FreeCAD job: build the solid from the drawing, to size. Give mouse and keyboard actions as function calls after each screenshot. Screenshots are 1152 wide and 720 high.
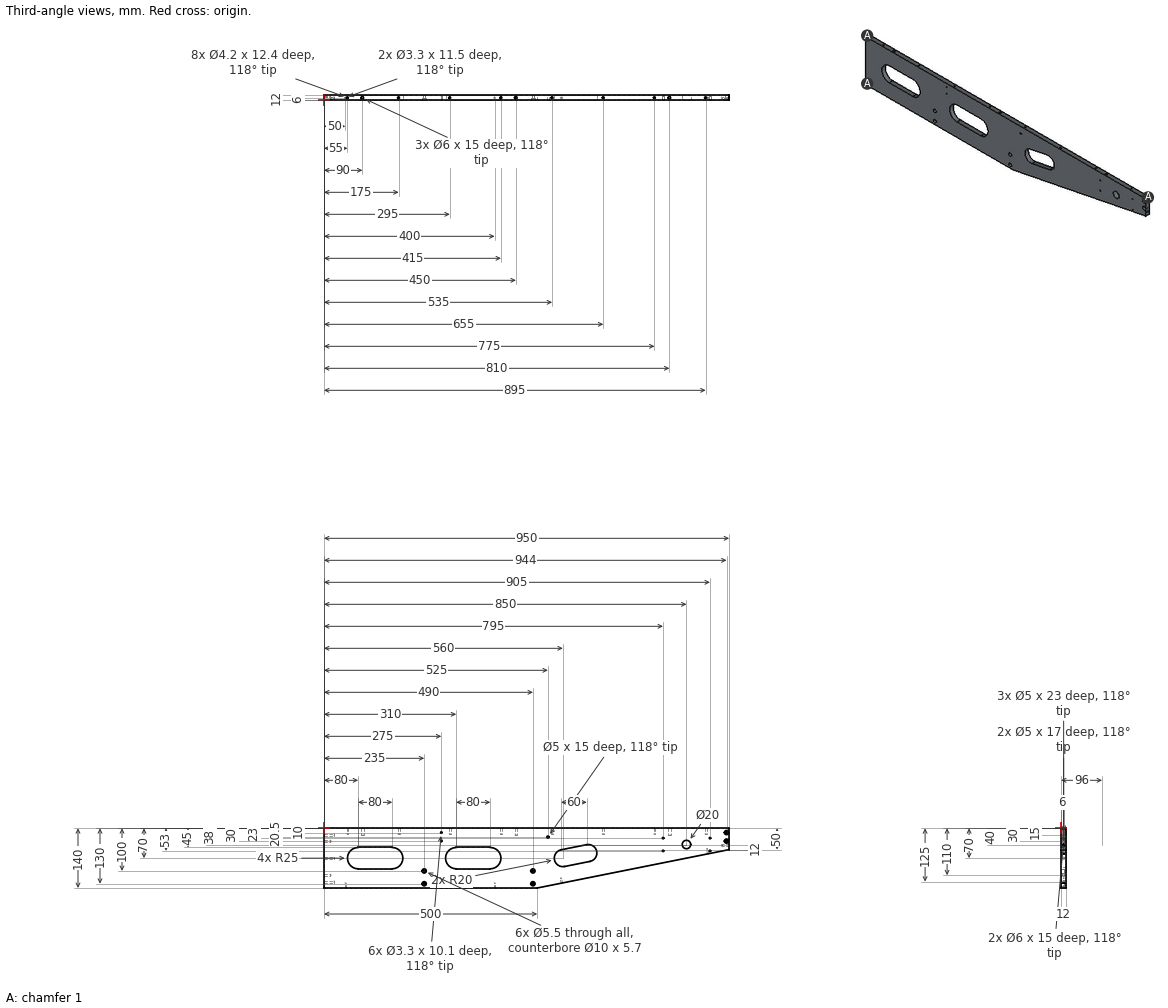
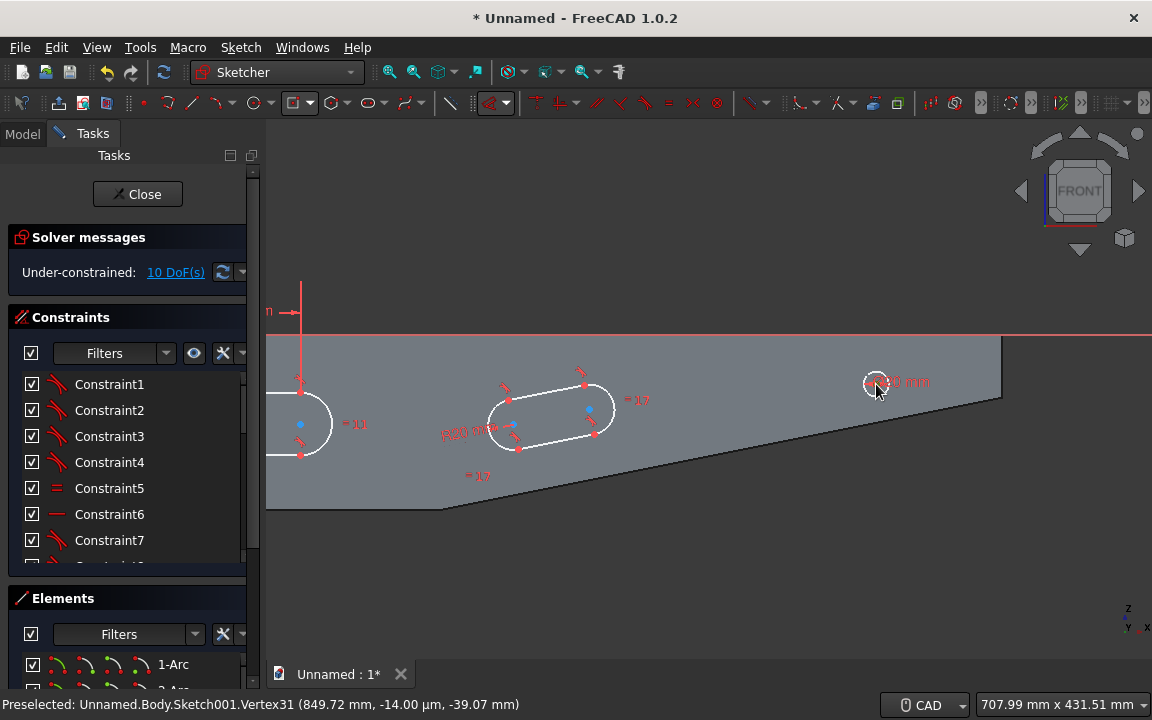
key(i)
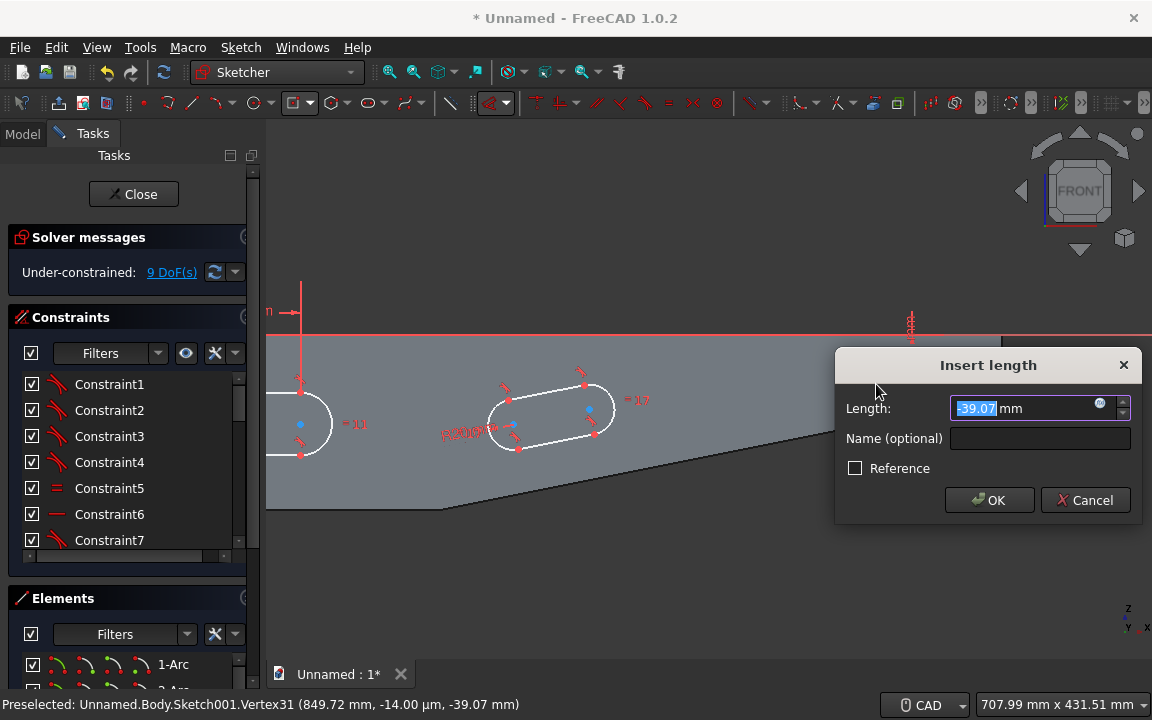
text(-38)
key(Return)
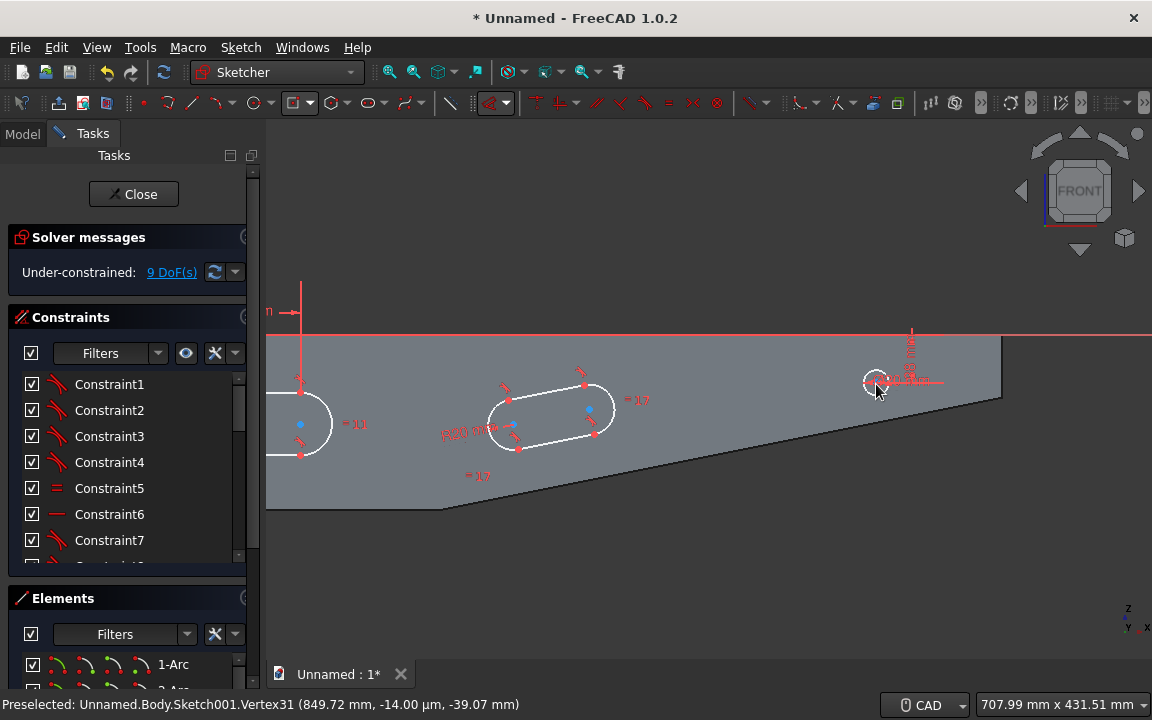
scroll(877, 384, down, 4)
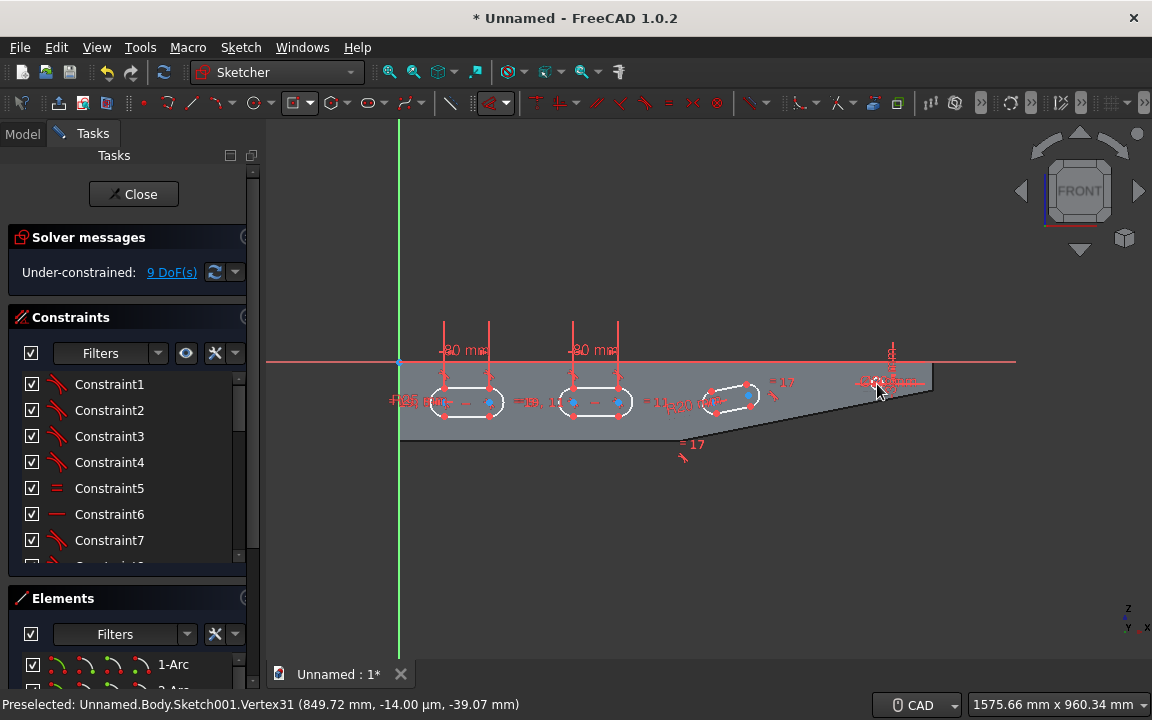
click(444, 388)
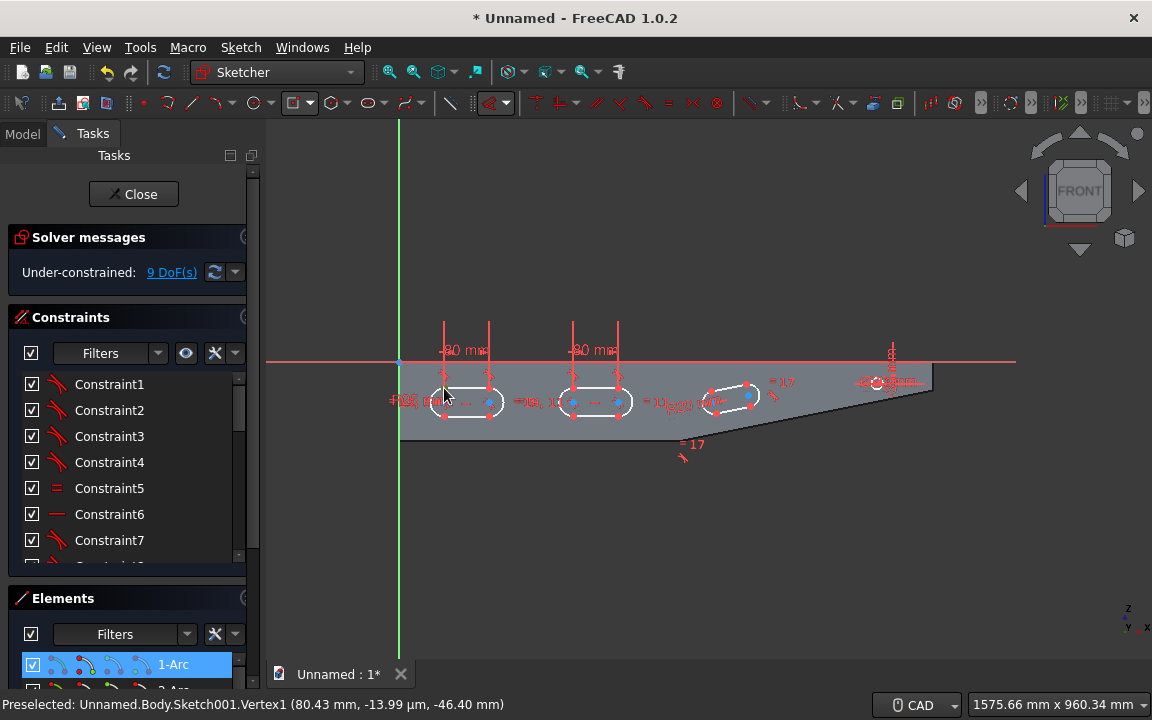
key(l)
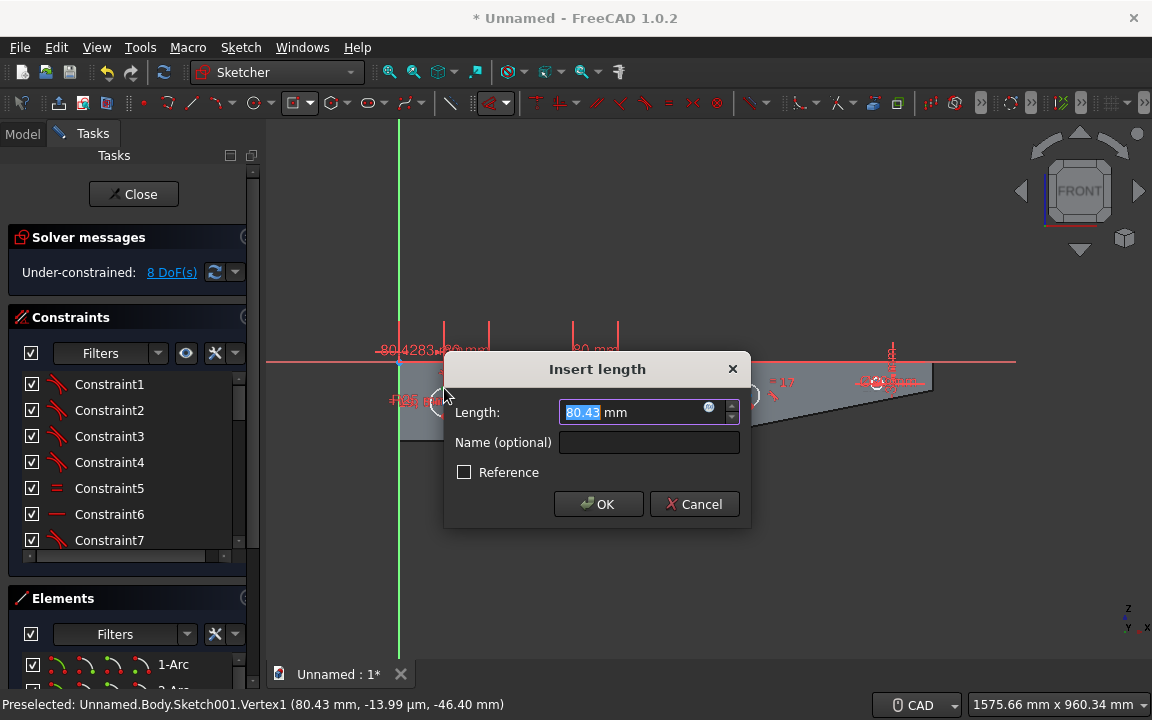
text(80)
key(Return)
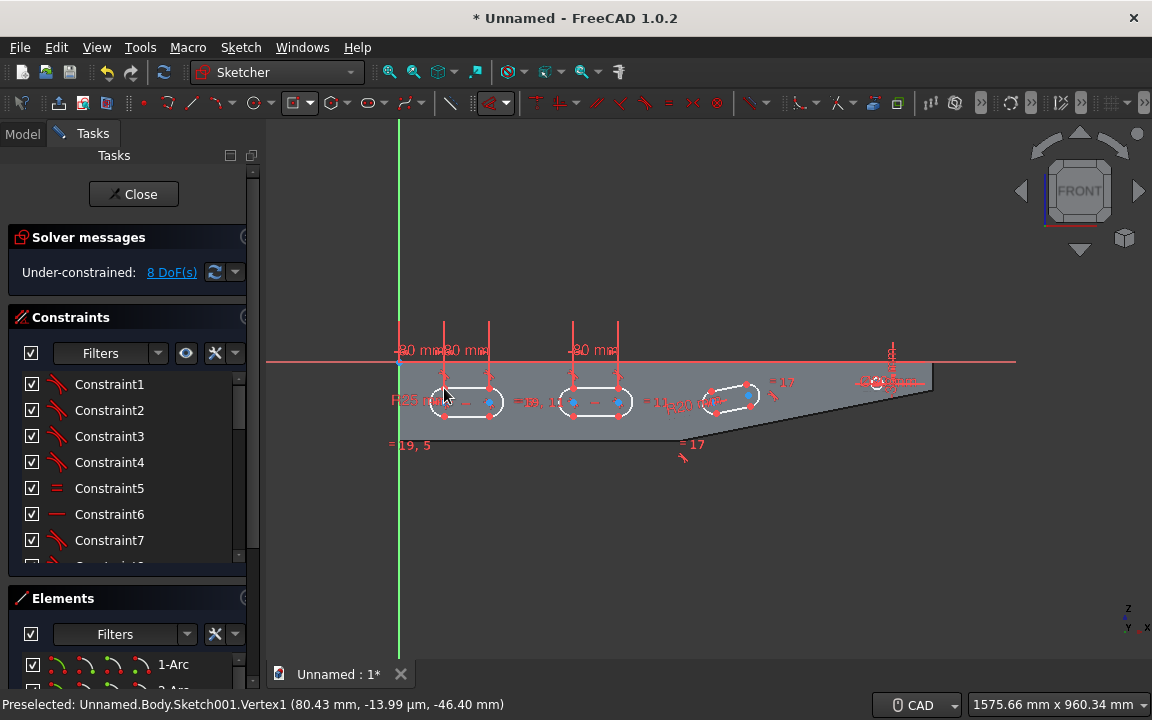
scroll(444, 388, up, 3)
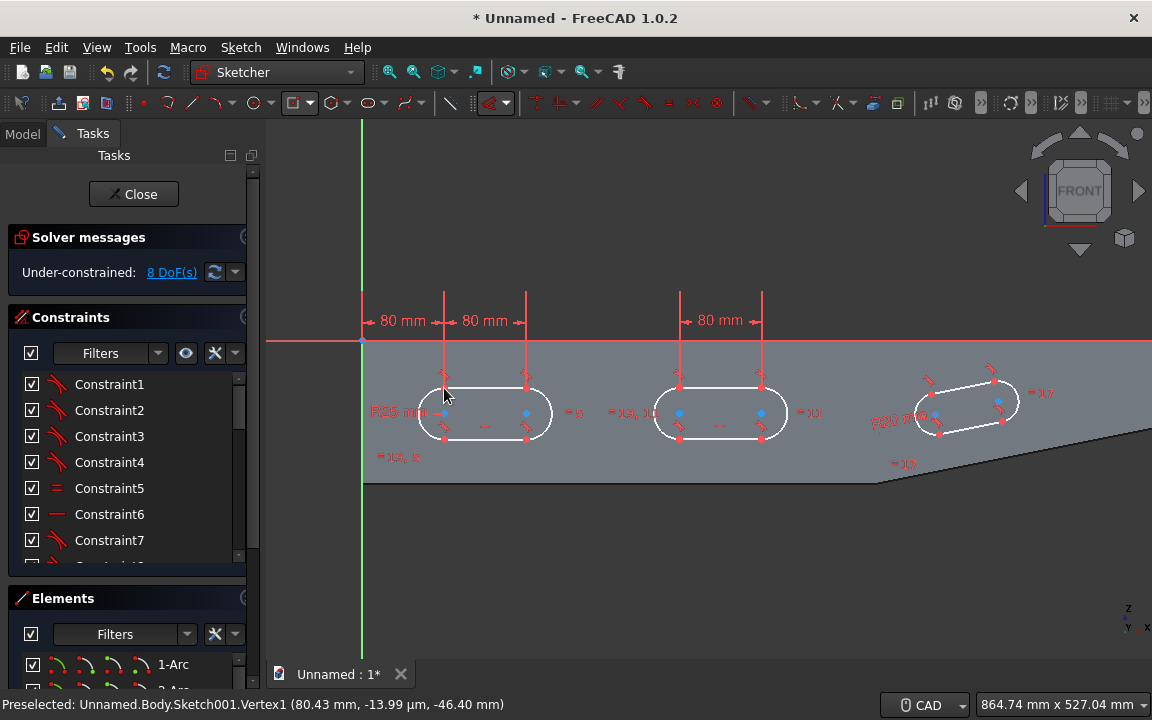
click(444, 388)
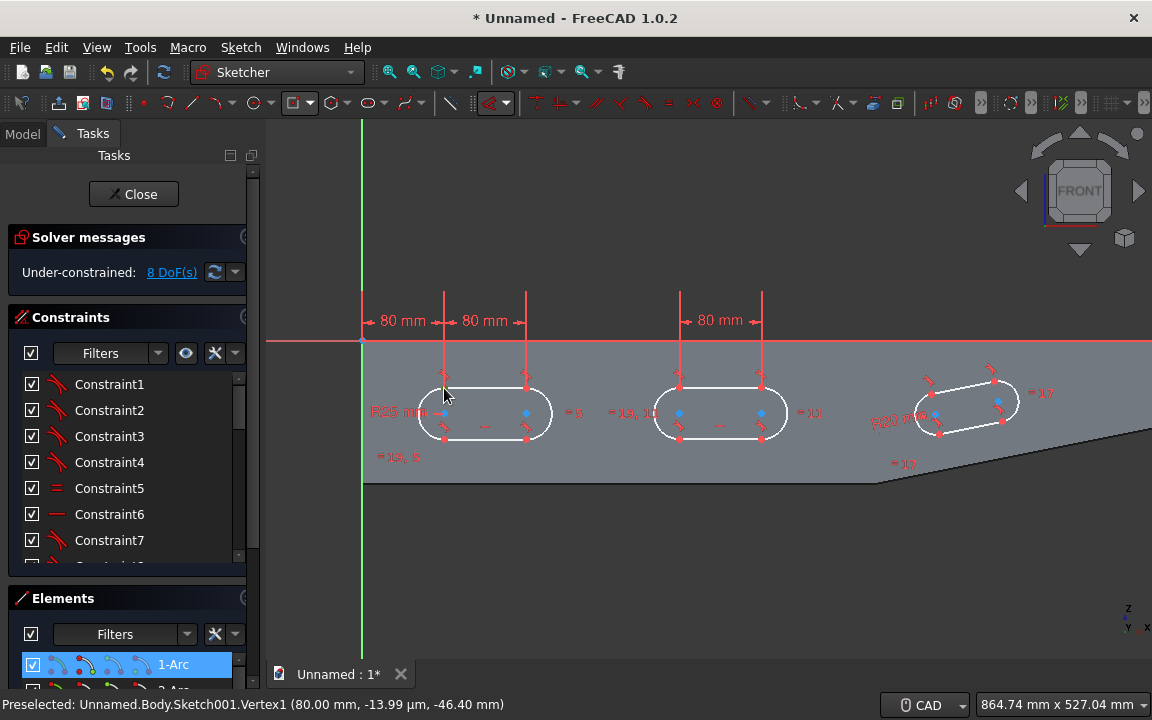
key(i)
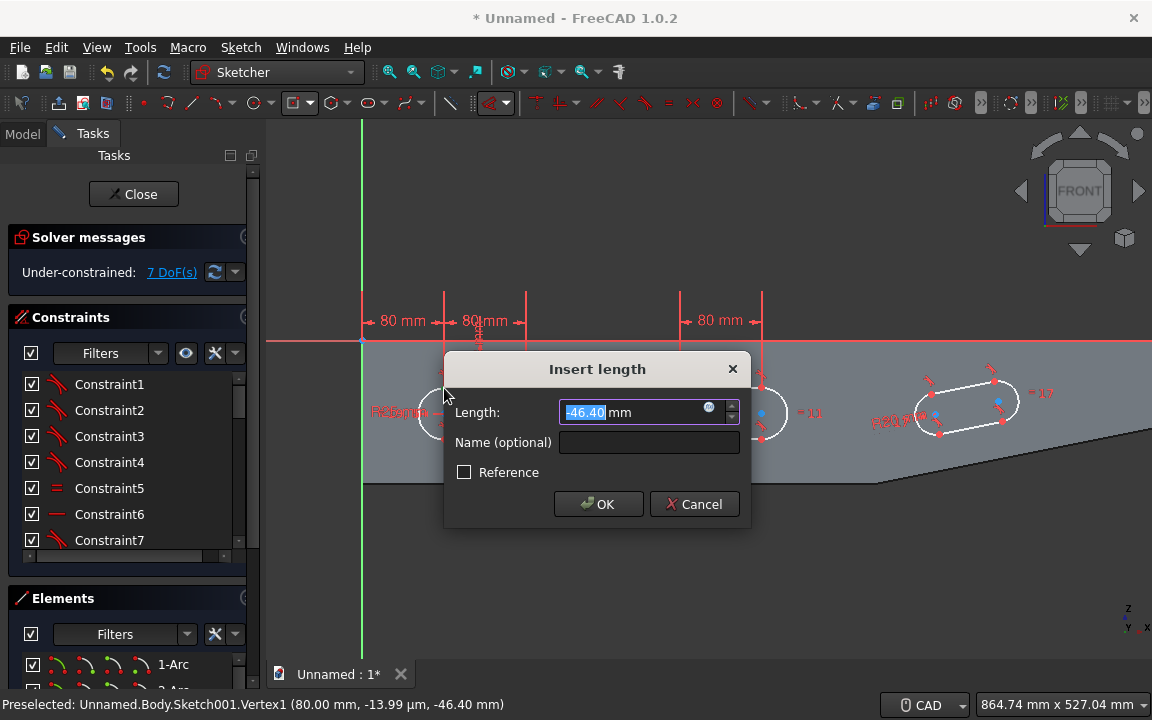
text(-45)
key(Return)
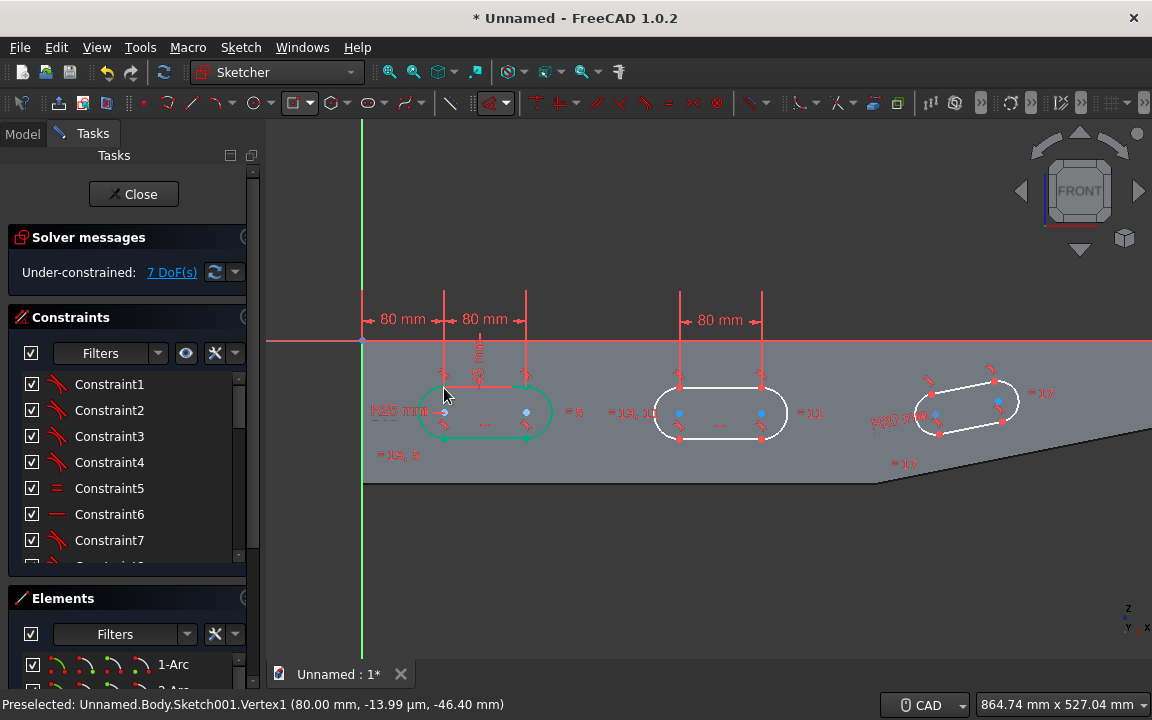
click(680, 388)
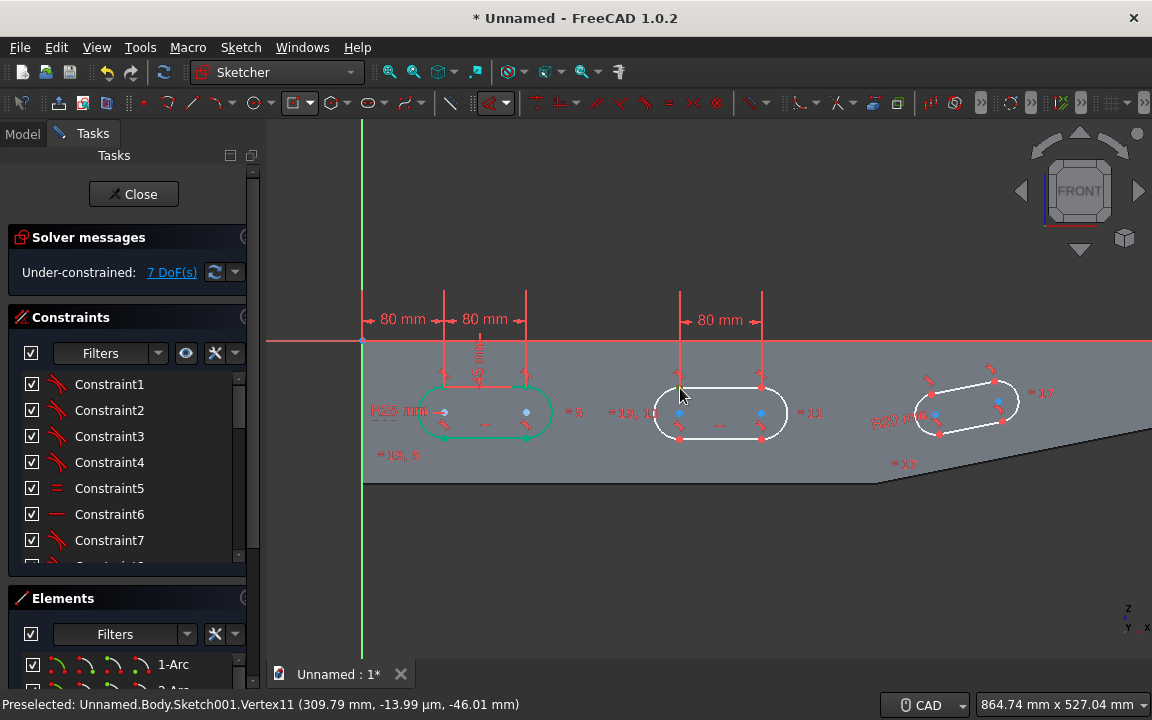
click(508, 104)